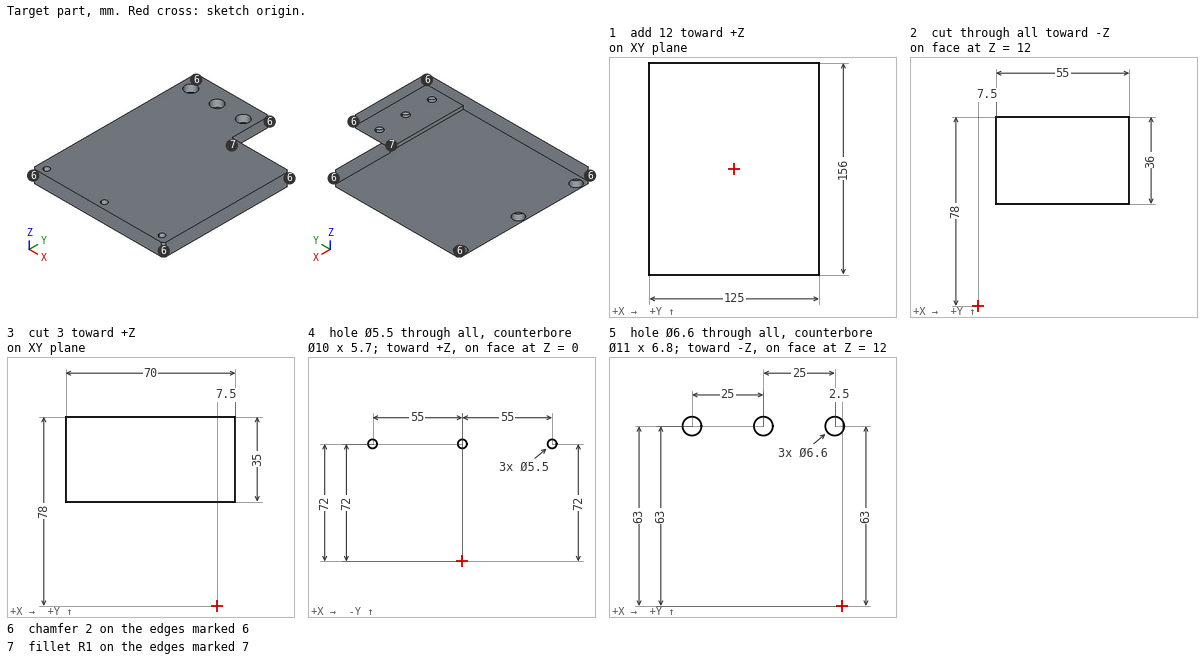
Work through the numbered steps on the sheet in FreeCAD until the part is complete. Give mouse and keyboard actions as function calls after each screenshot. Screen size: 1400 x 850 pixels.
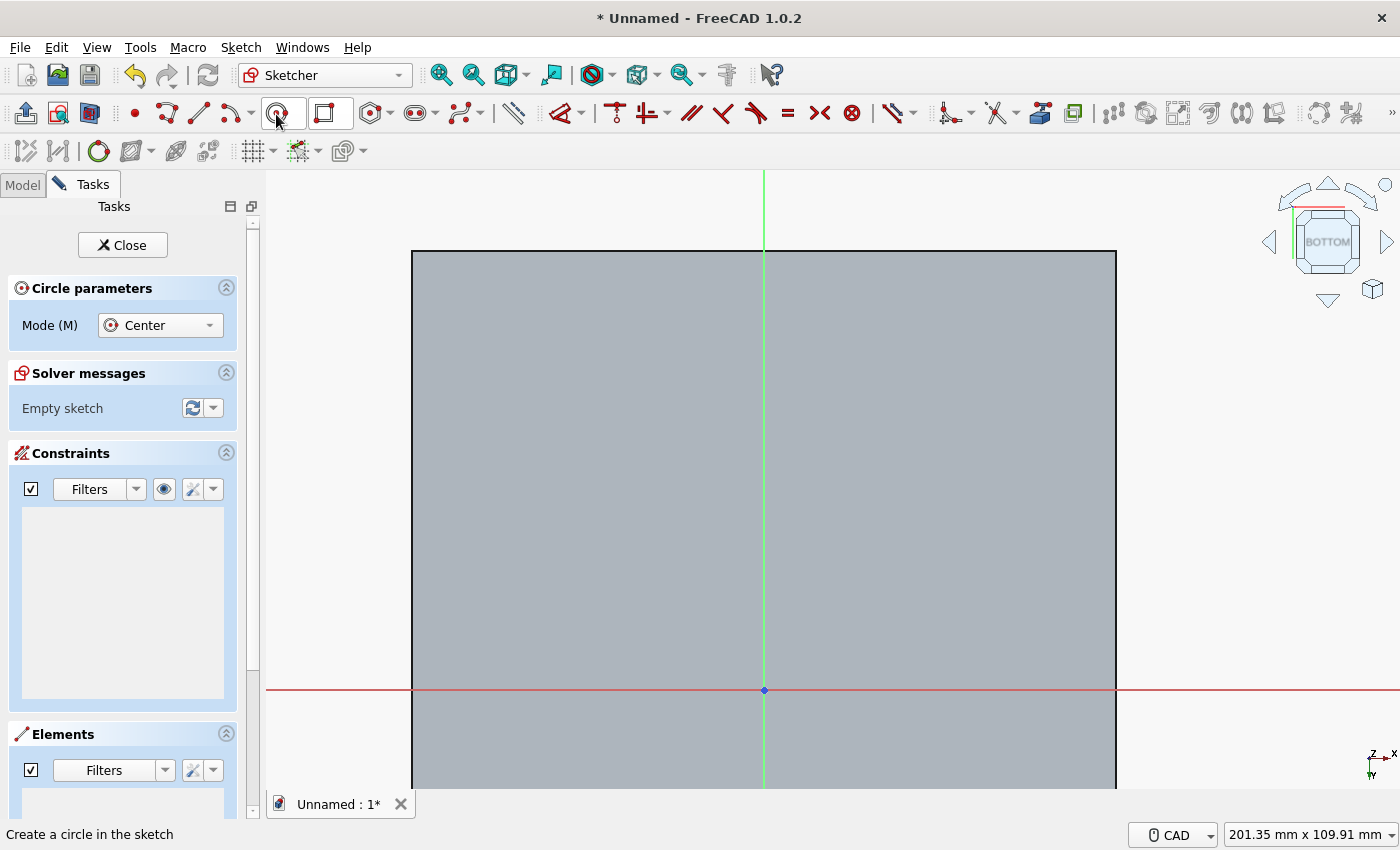
scroll(1074, 285, up, 2)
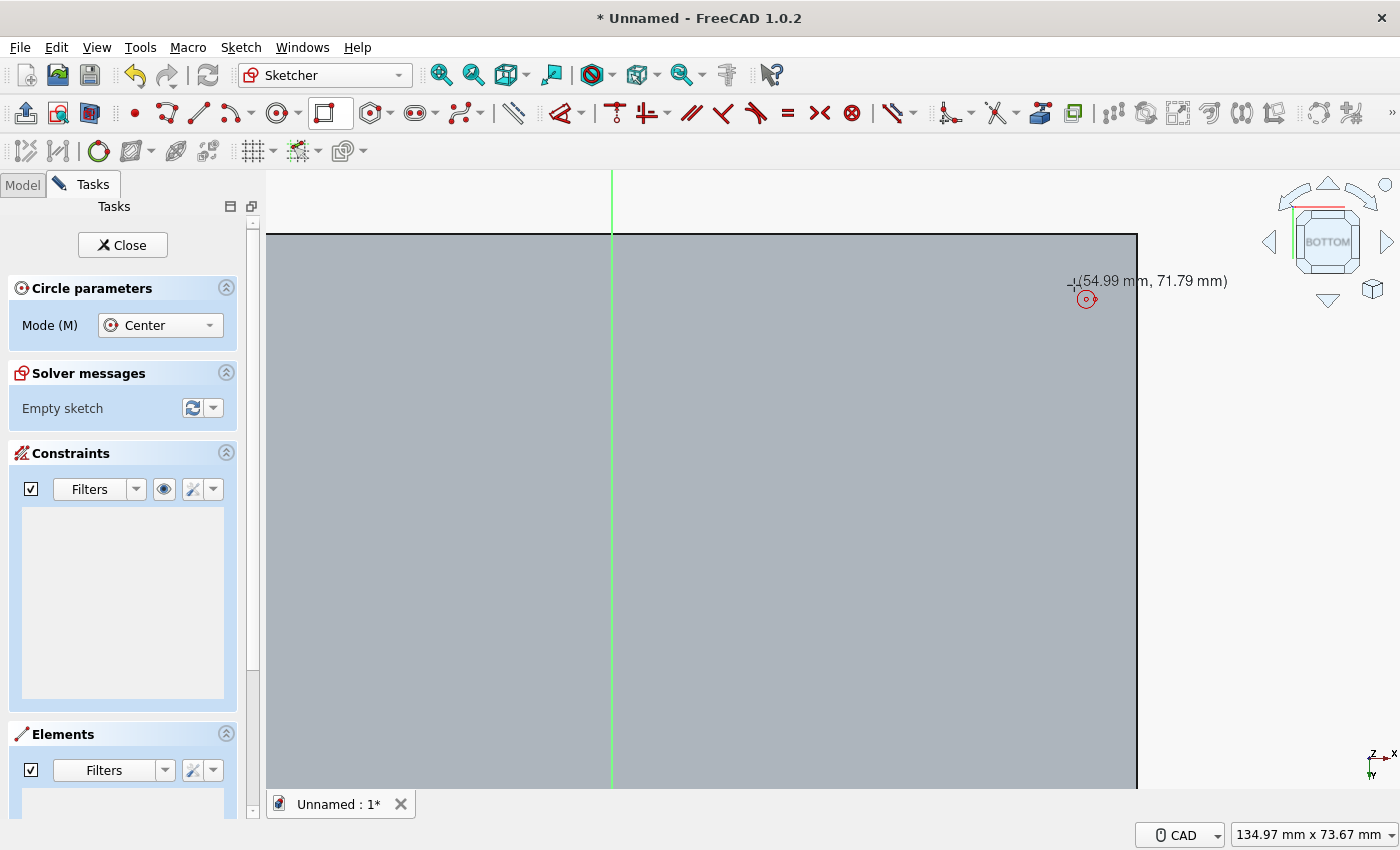
click(1074, 285)
move(1090, 268)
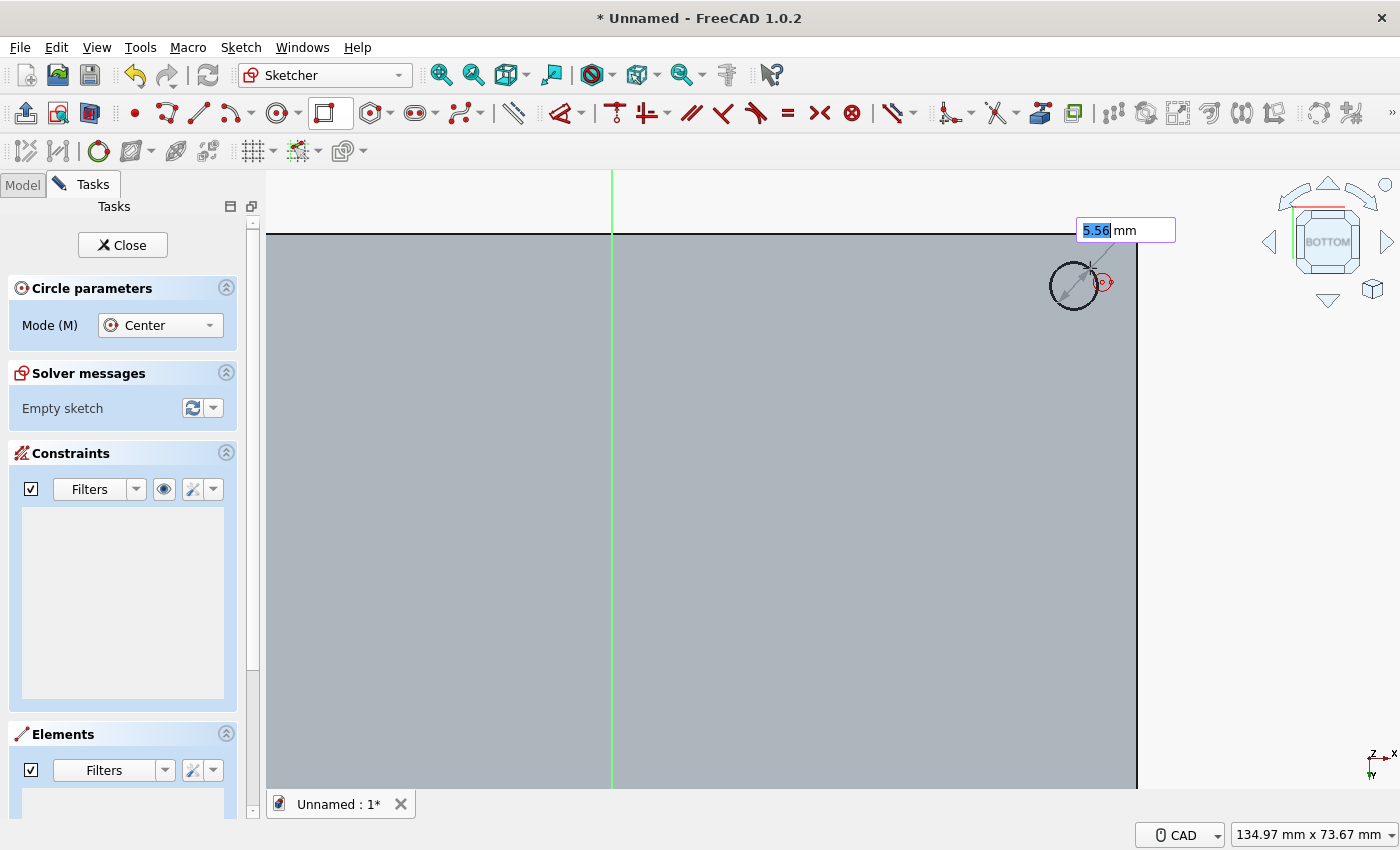
text(5.5)
key(Return)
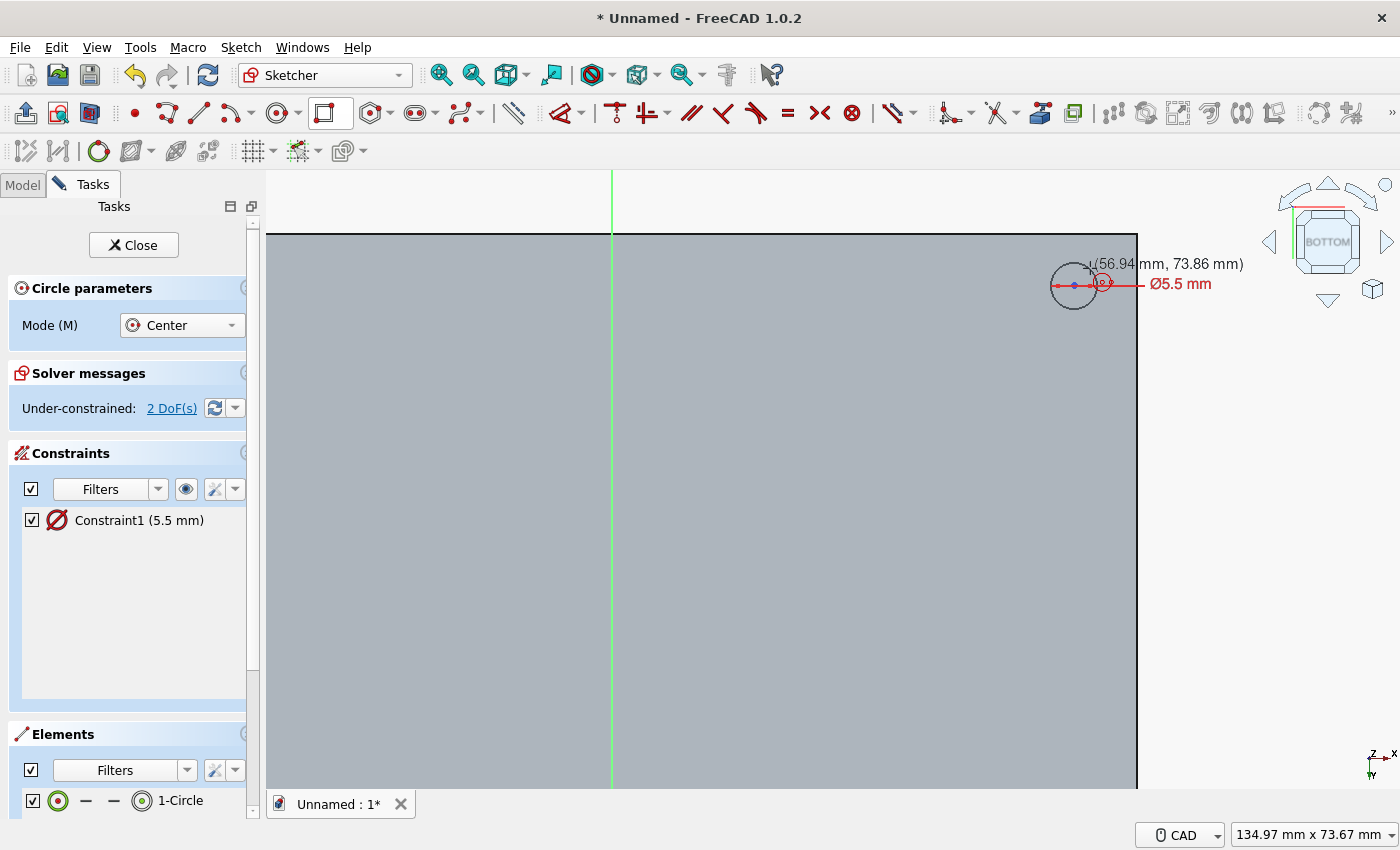
click(612, 285)
move(628, 268)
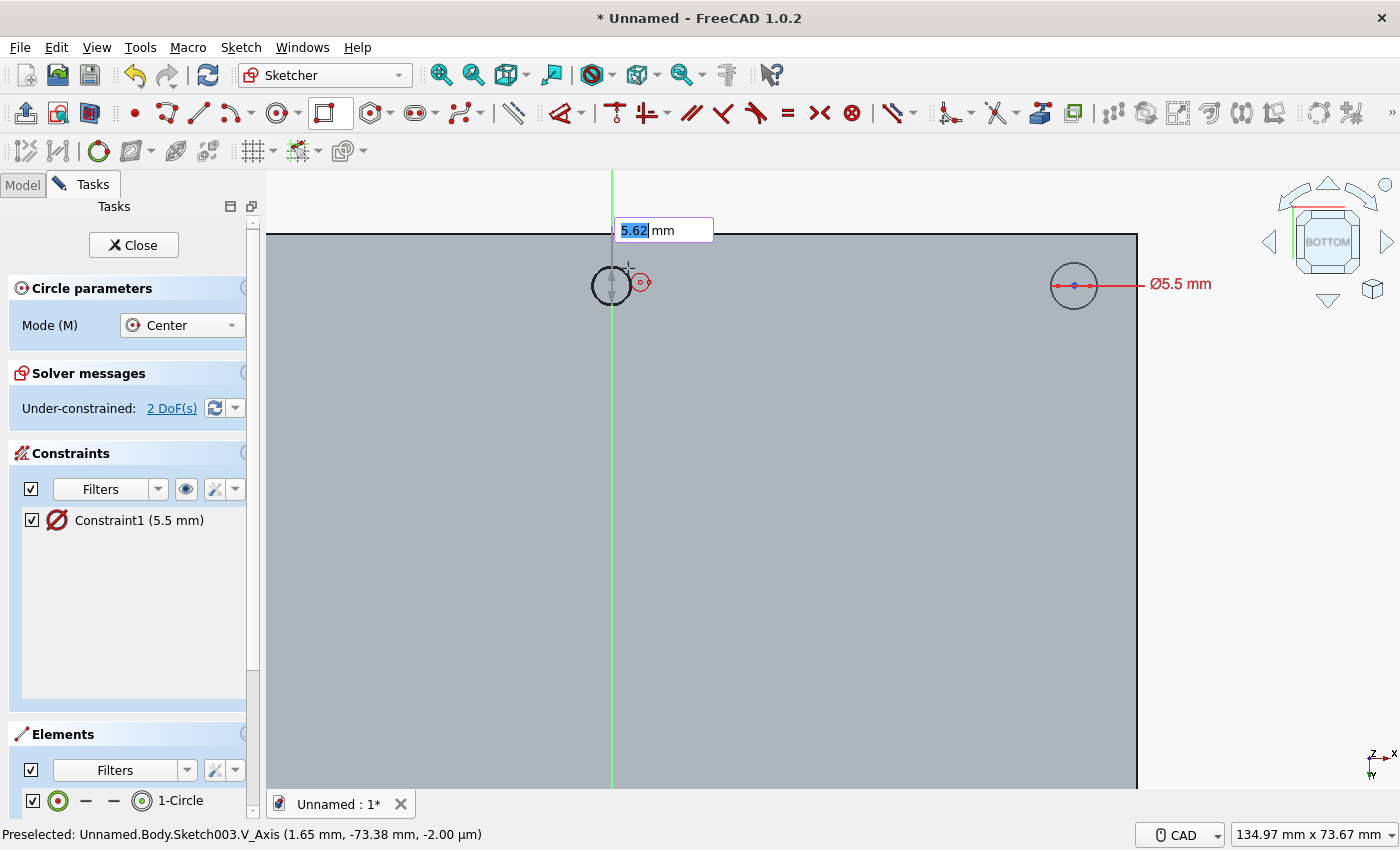
text(5.5)
key(Return)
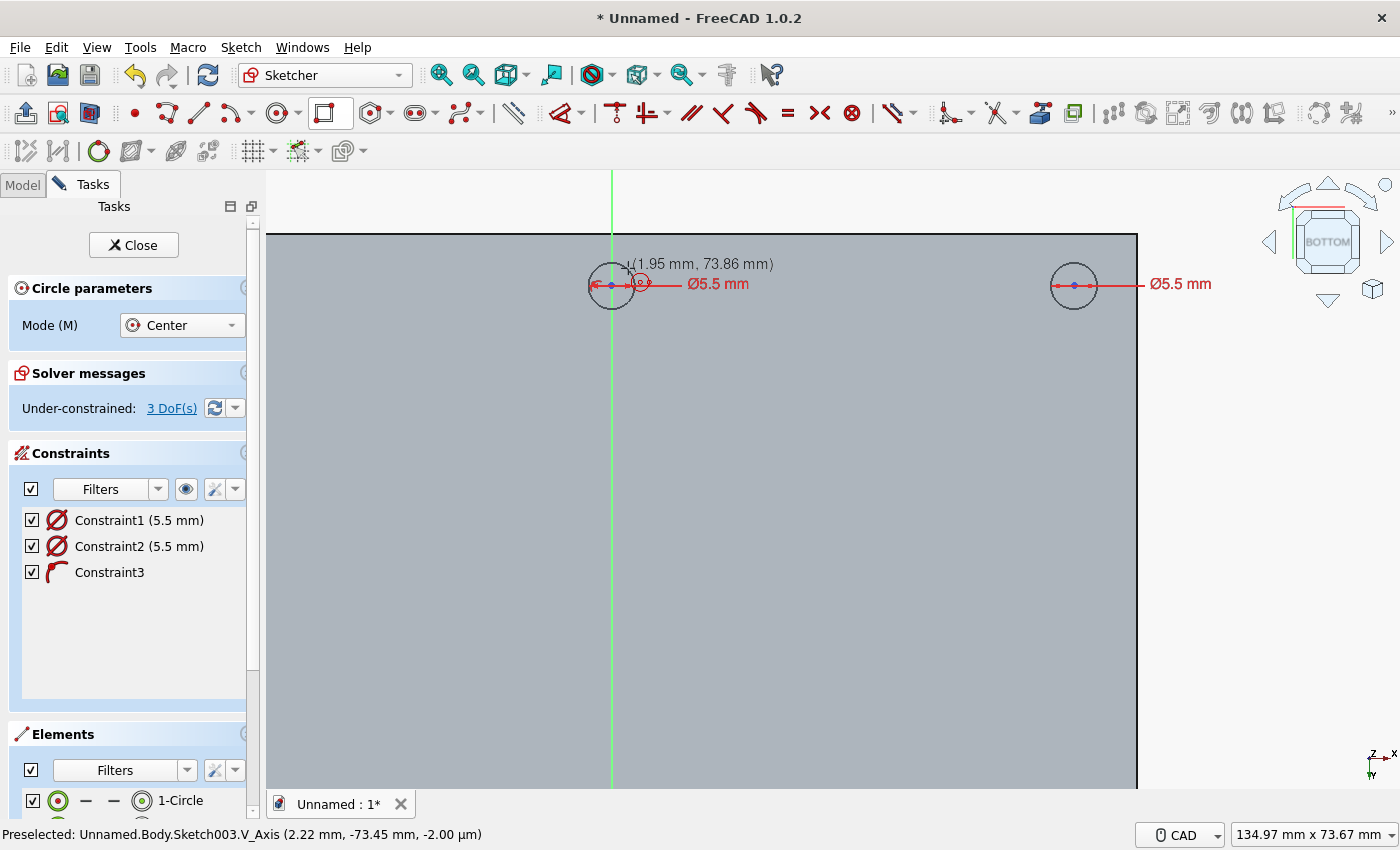
scroll(1075, 284, down, 2)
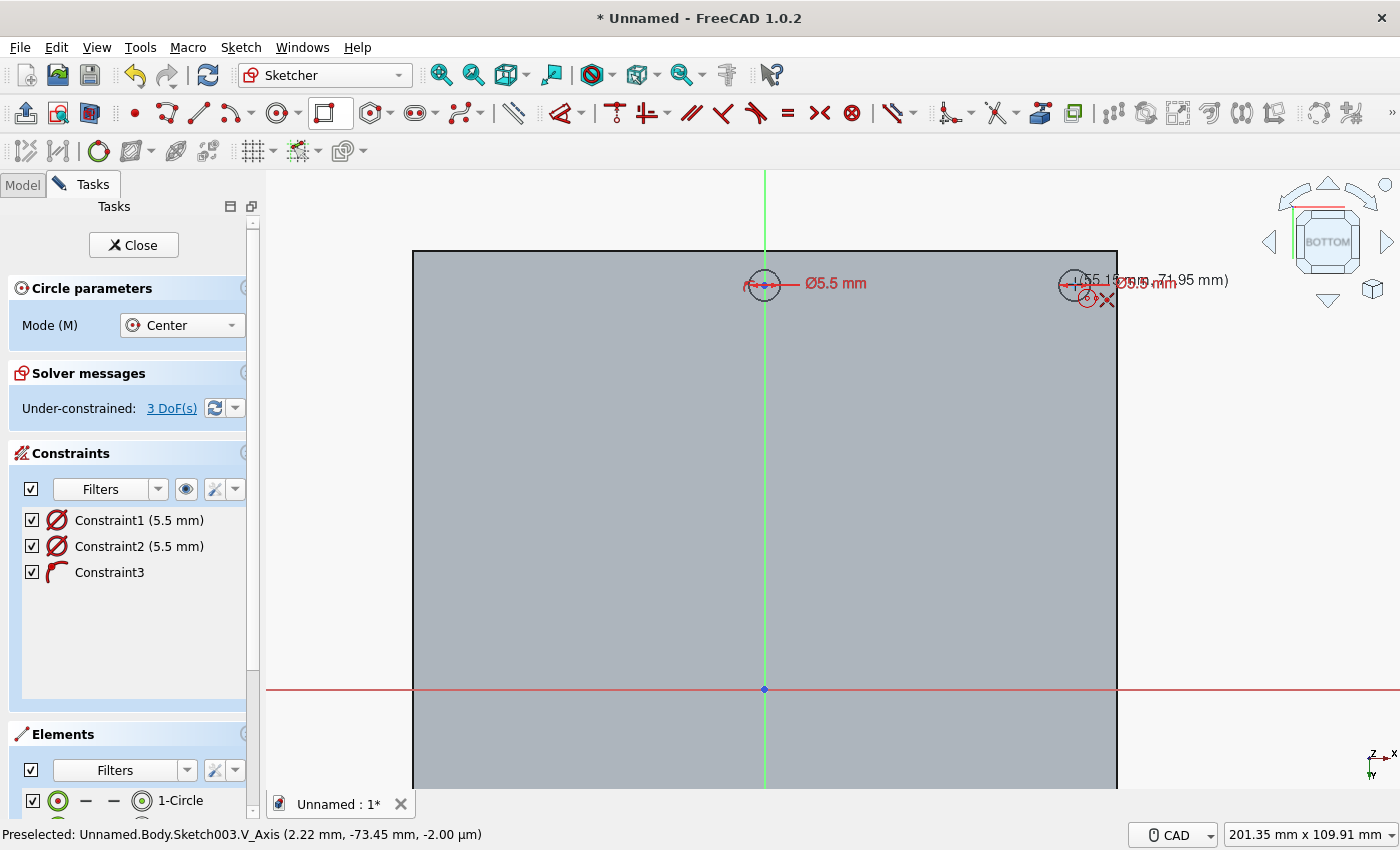
scroll(455, 284, up, 2)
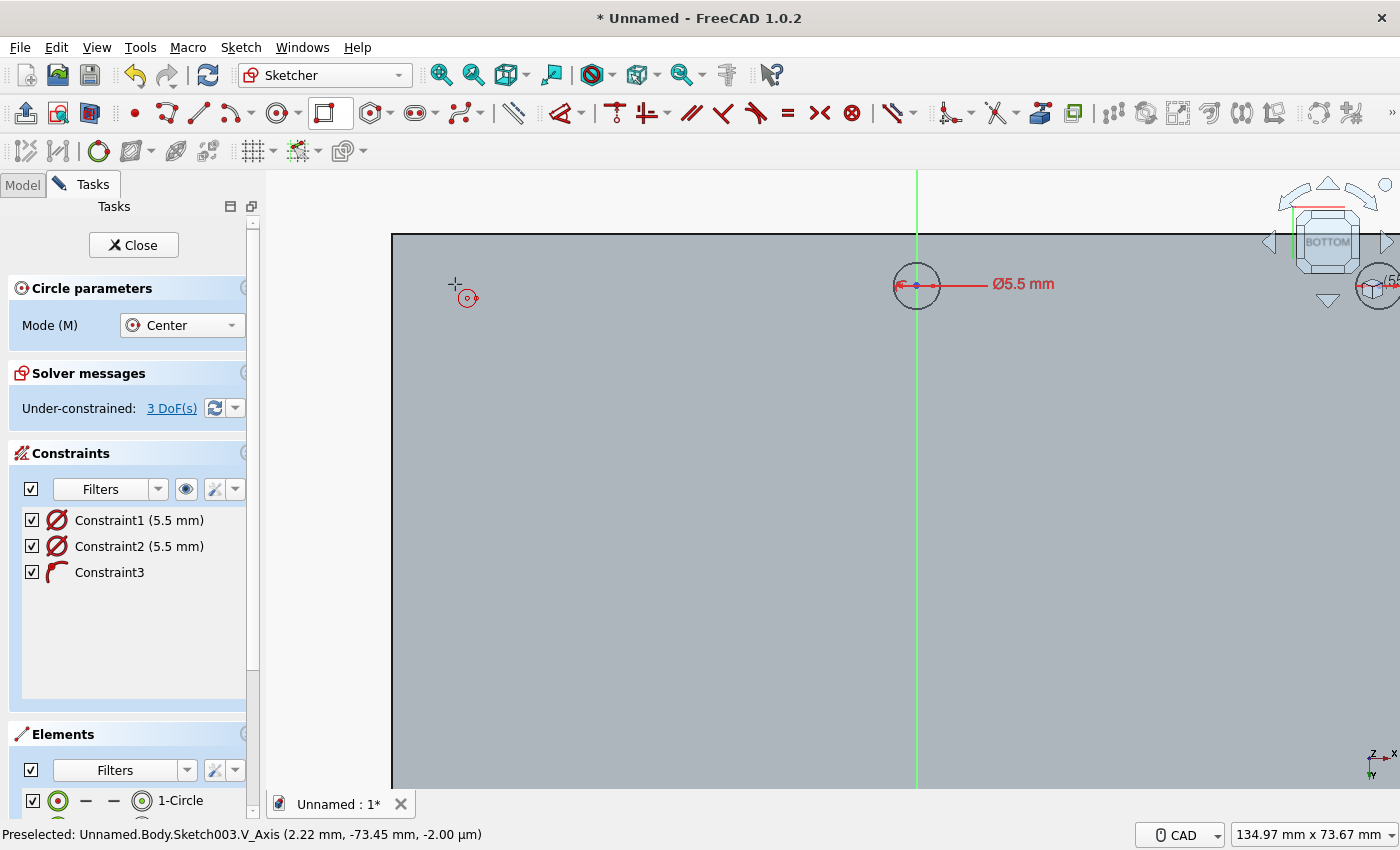
click(455, 285)
move(471, 268)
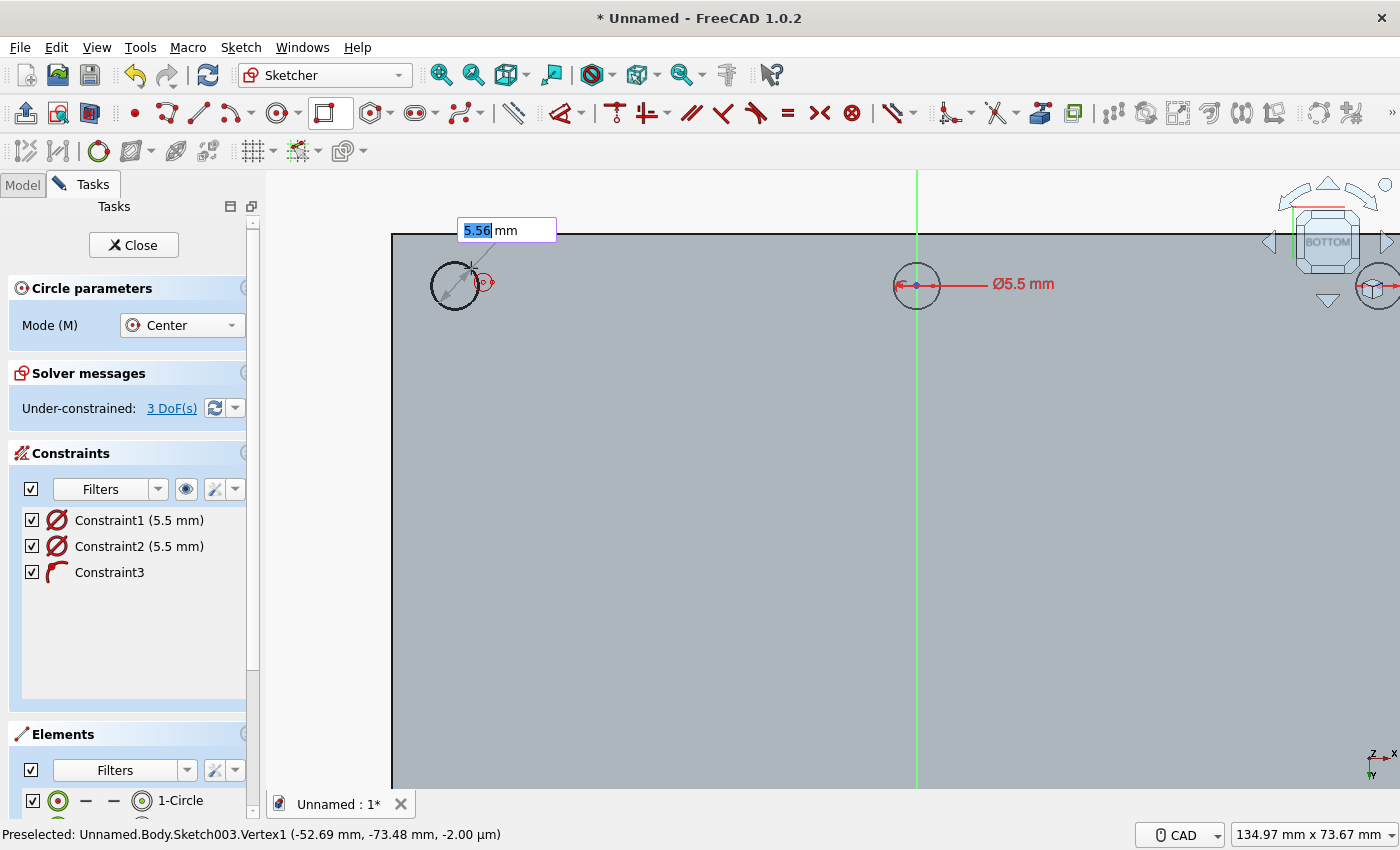
text(5.5)
key(Return)
key(Escape)